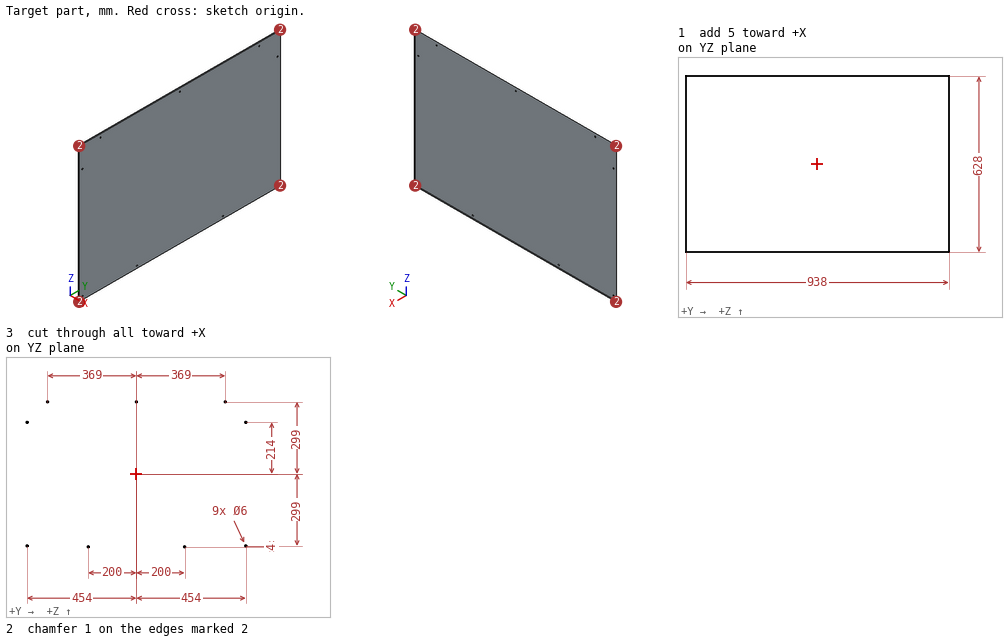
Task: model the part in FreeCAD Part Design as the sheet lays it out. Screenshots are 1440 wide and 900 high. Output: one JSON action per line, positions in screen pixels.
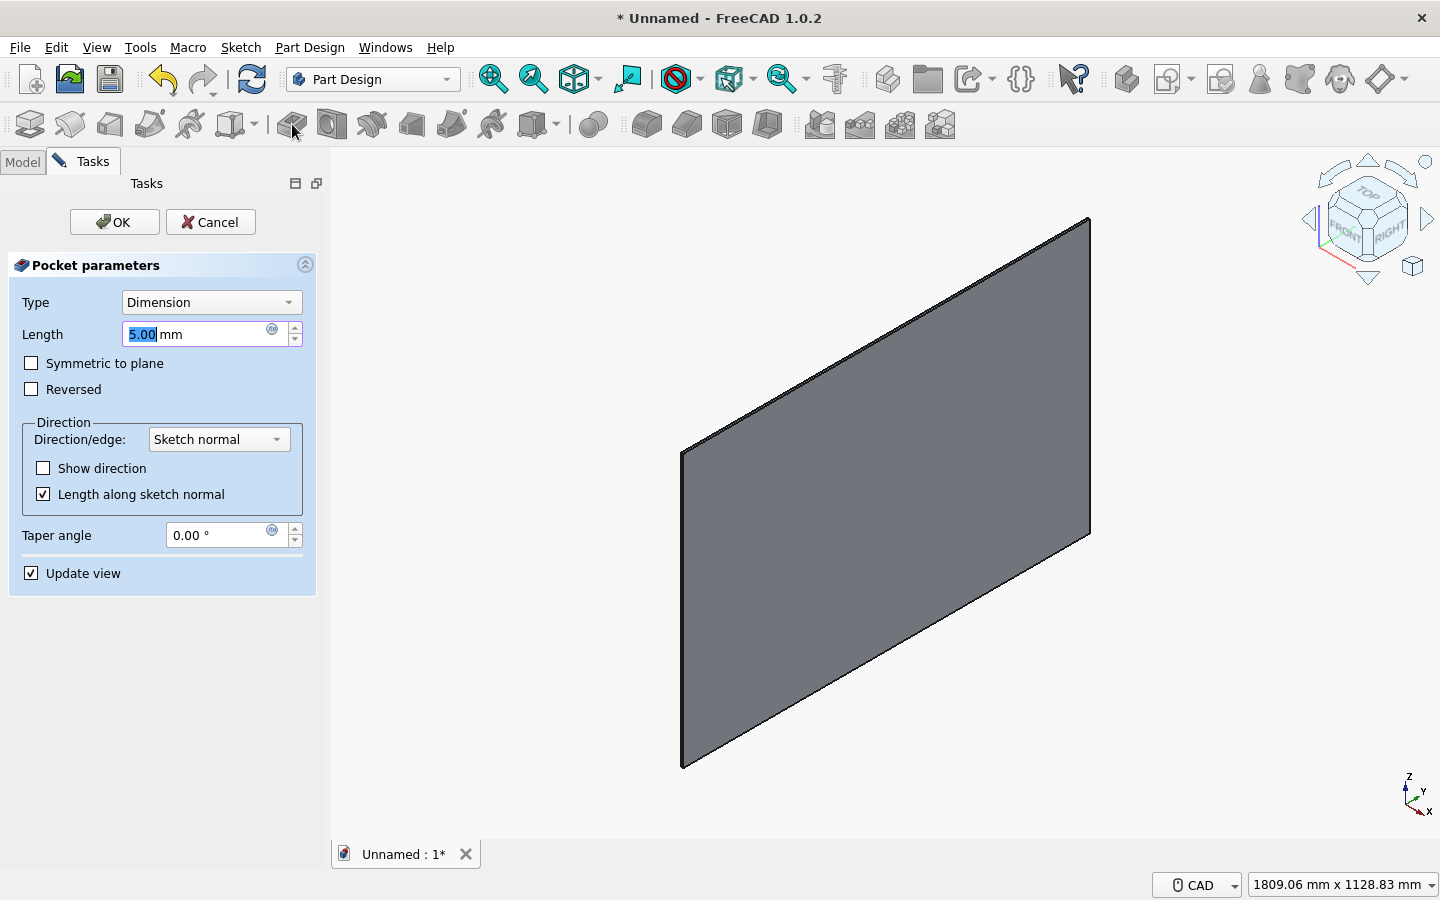
{"action": "left_click", "coordinate": [212, 302]}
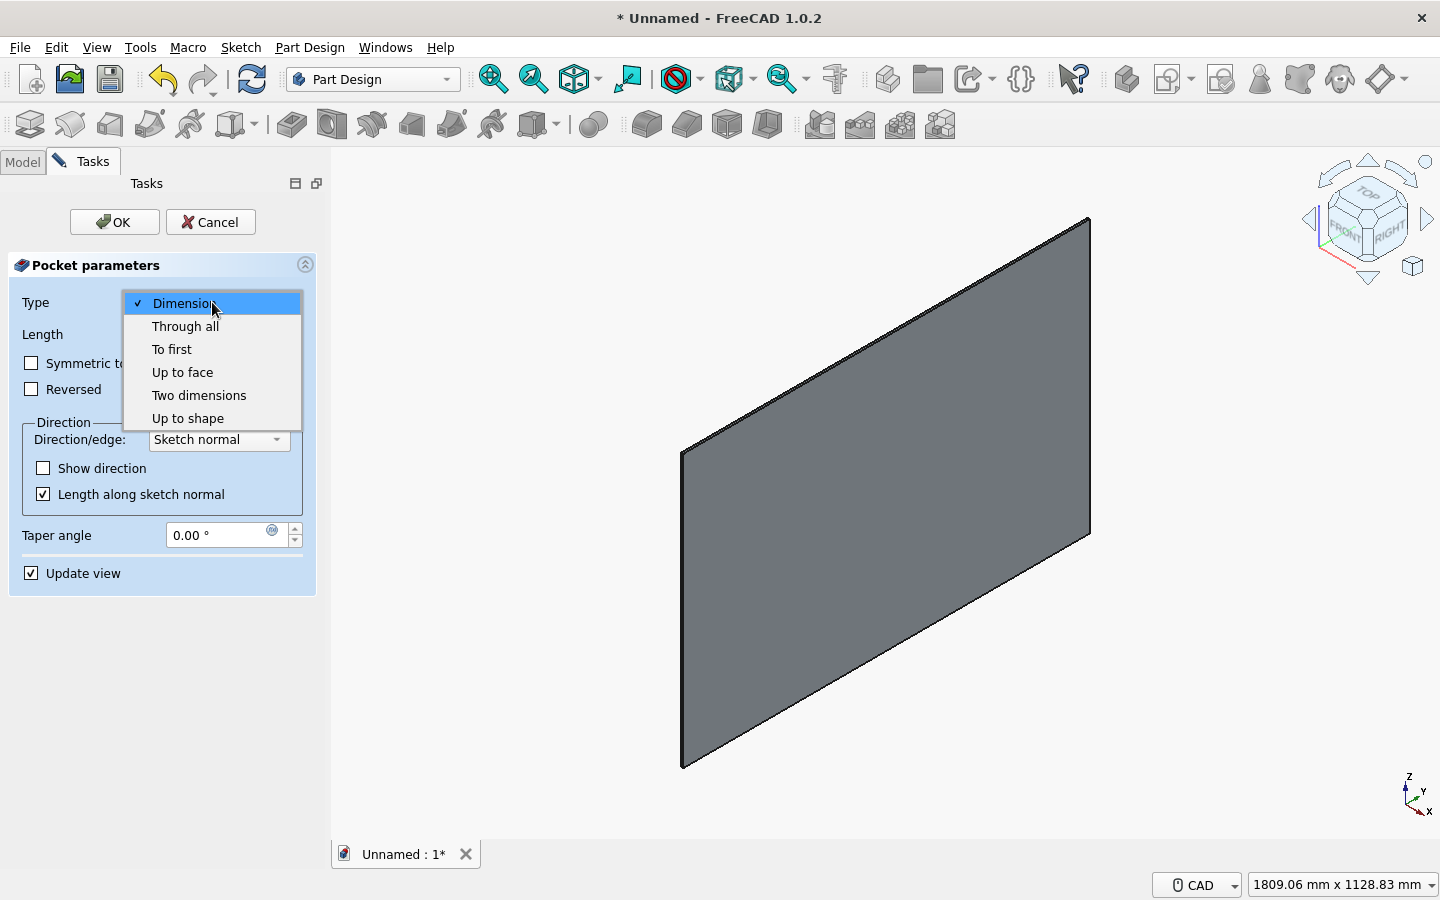
{"action": "left_click", "coordinate": [212, 326]}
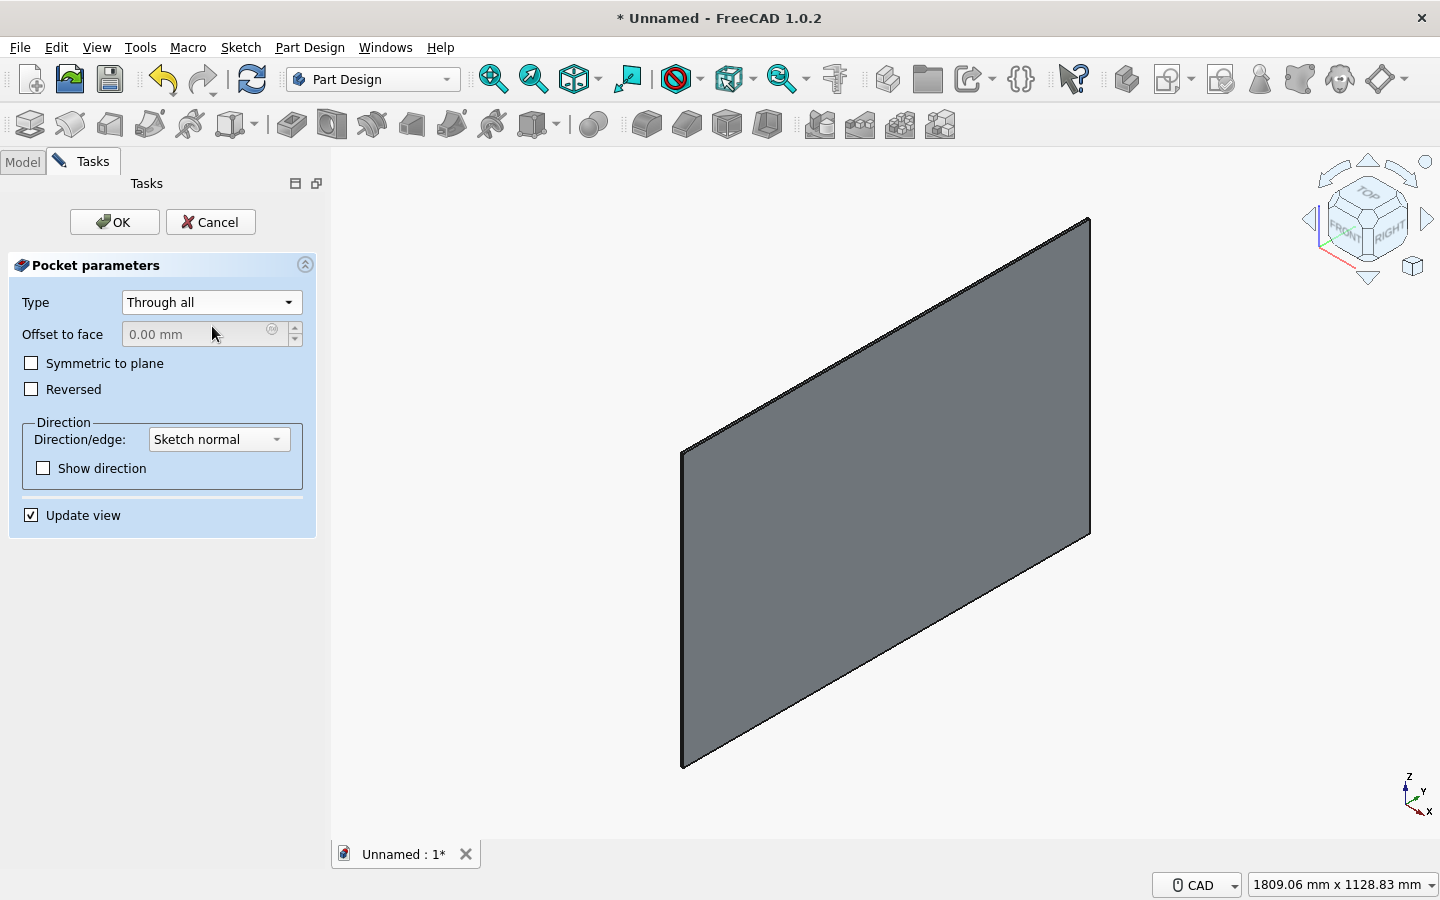
{"action": "left_click", "coordinate": [30, 389]}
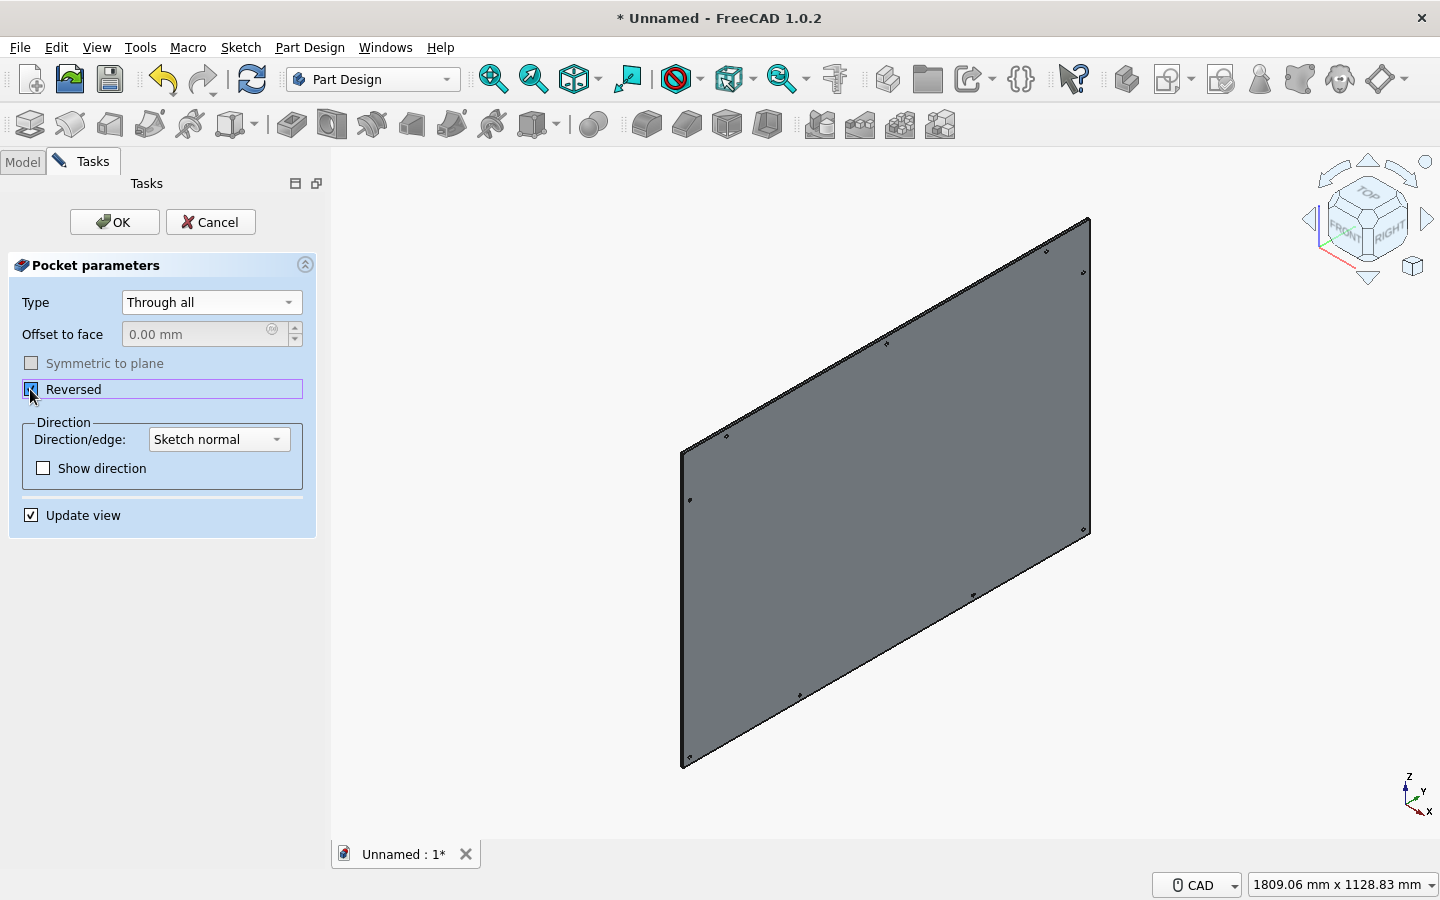
{"action": "left_click", "coordinate": [115, 222]}